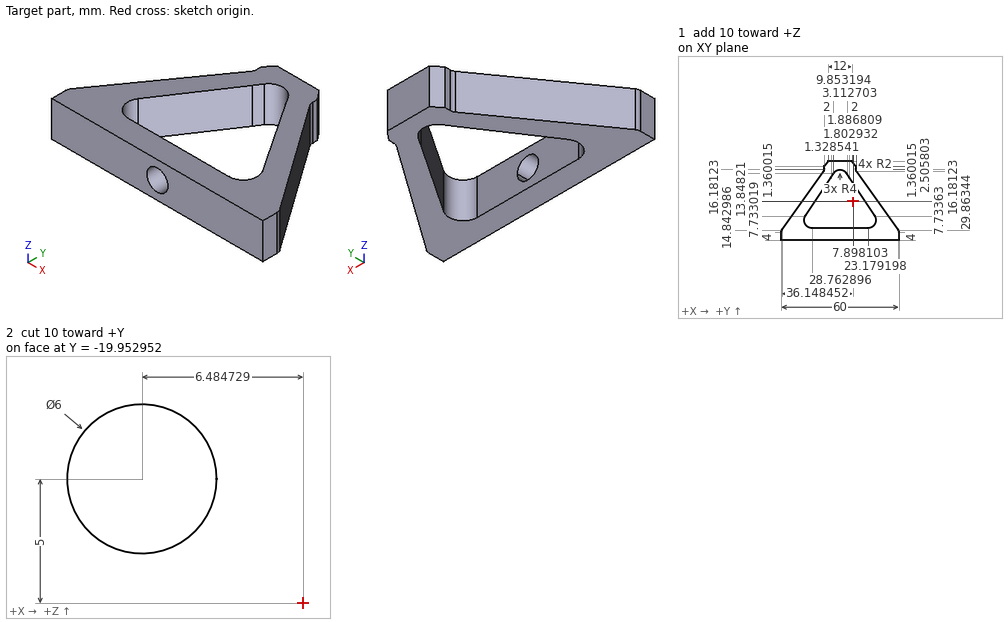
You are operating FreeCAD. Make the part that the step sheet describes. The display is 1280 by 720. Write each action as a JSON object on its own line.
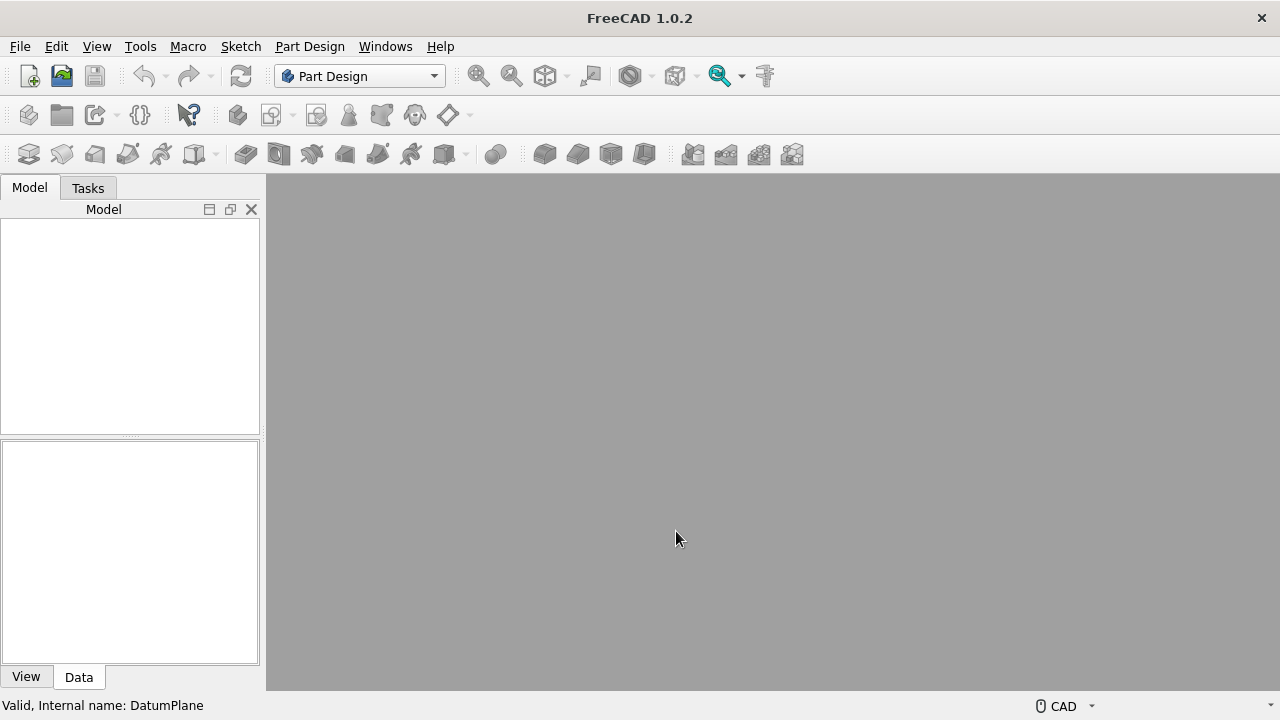
{"action": "left_click", "coordinate": [29, 76]}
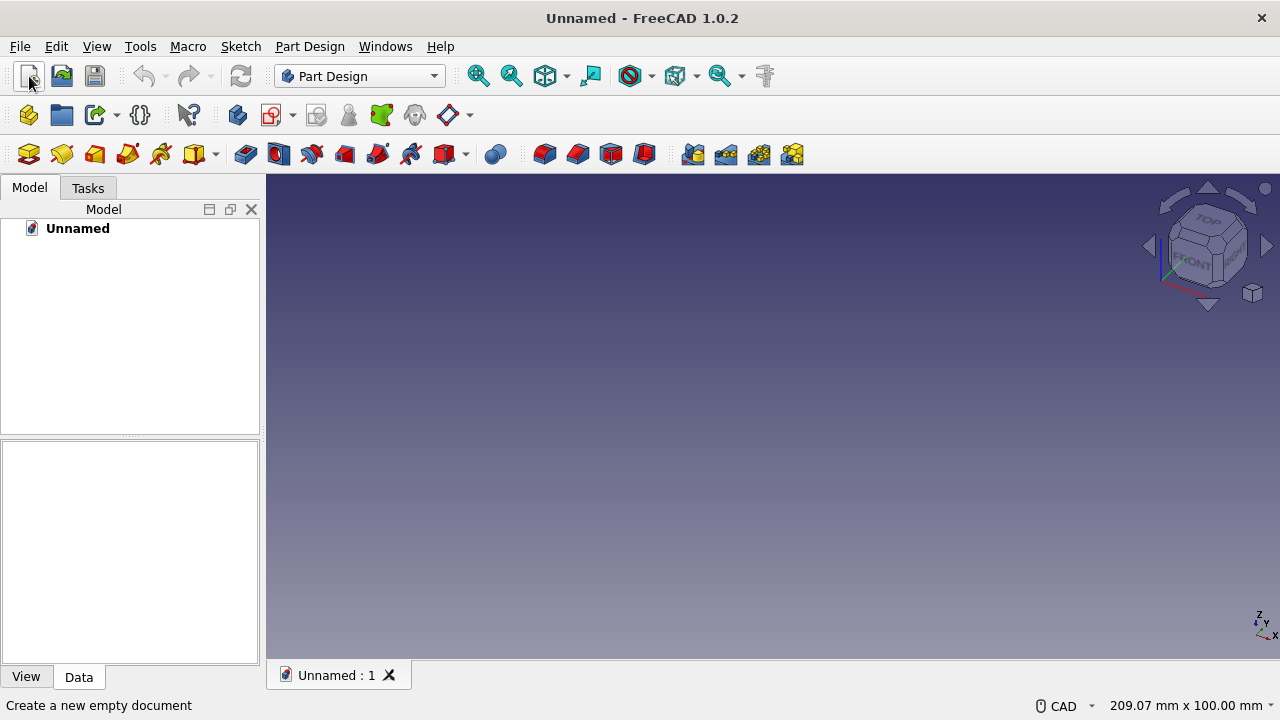
{"action": "left_click", "coordinate": [270, 116]}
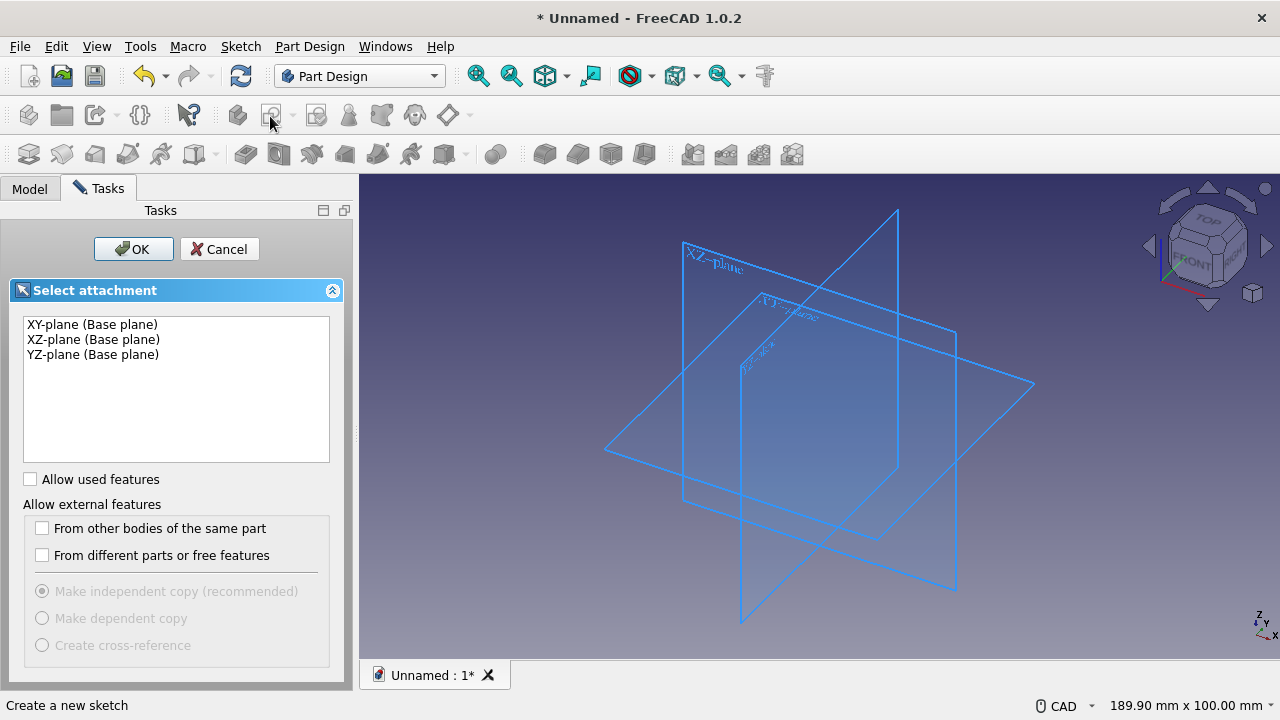
{"action": "left_click", "coordinate": [84, 324]}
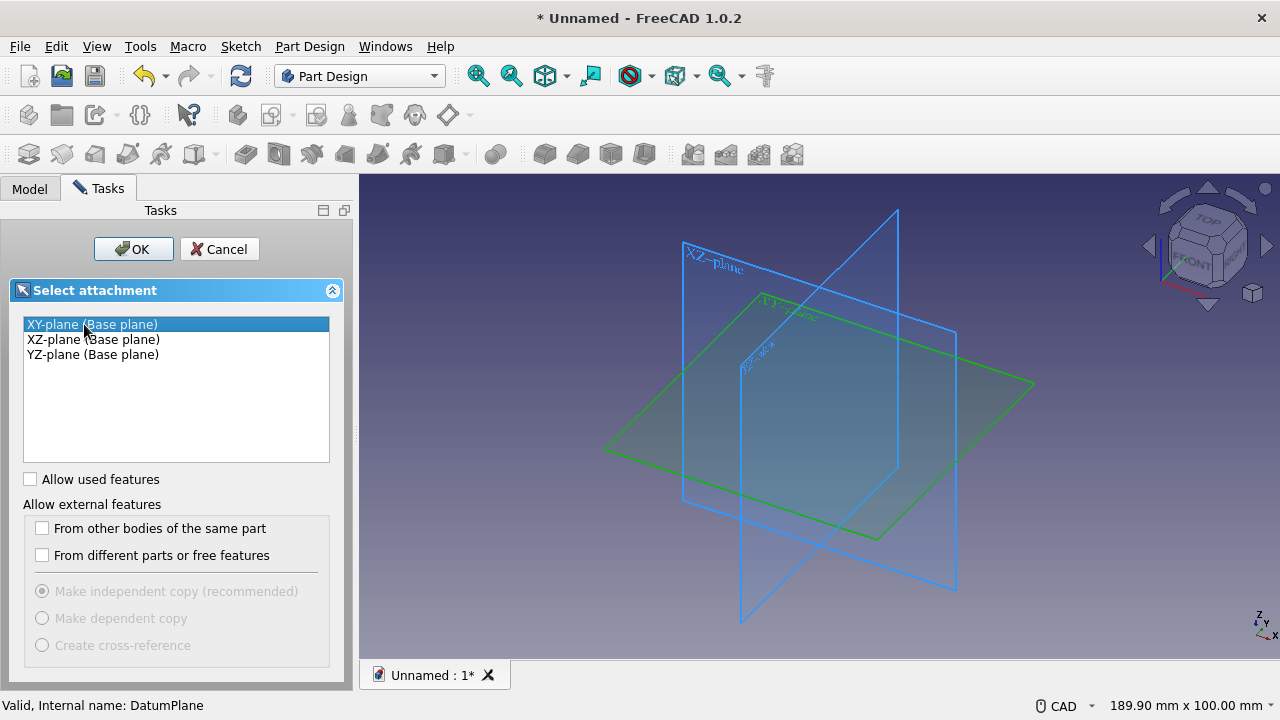
{"action": "left_click", "coordinate": [134, 249]}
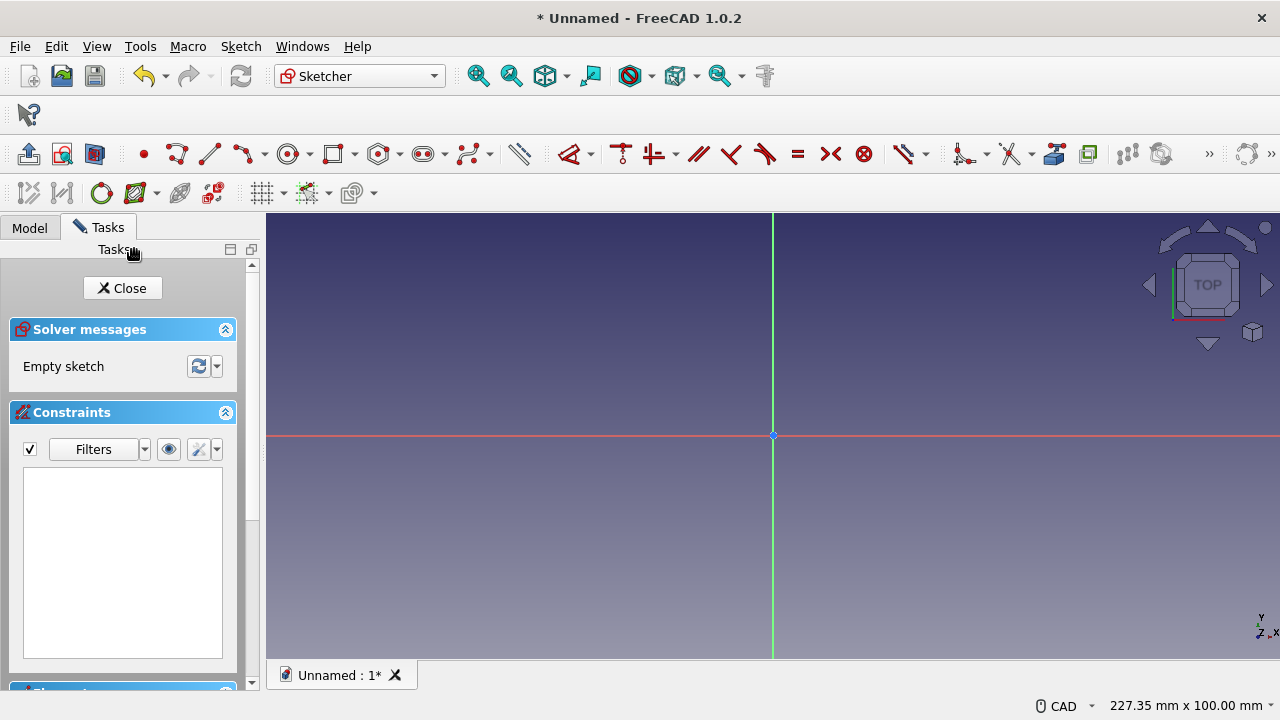
{"action": "scroll", "coordinate": [825, 435], "scroll_direction": "up", "scroll_amount": 2}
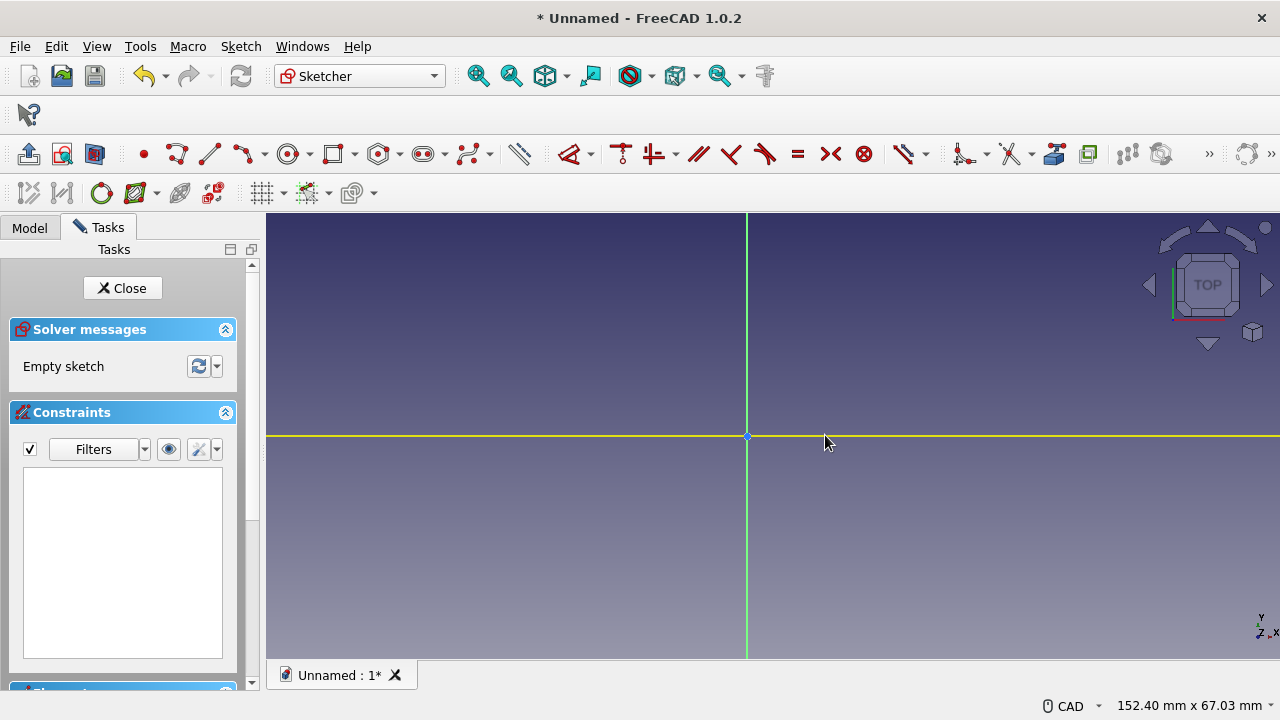
{"action": "left_click", "coordinate": [210, 154]}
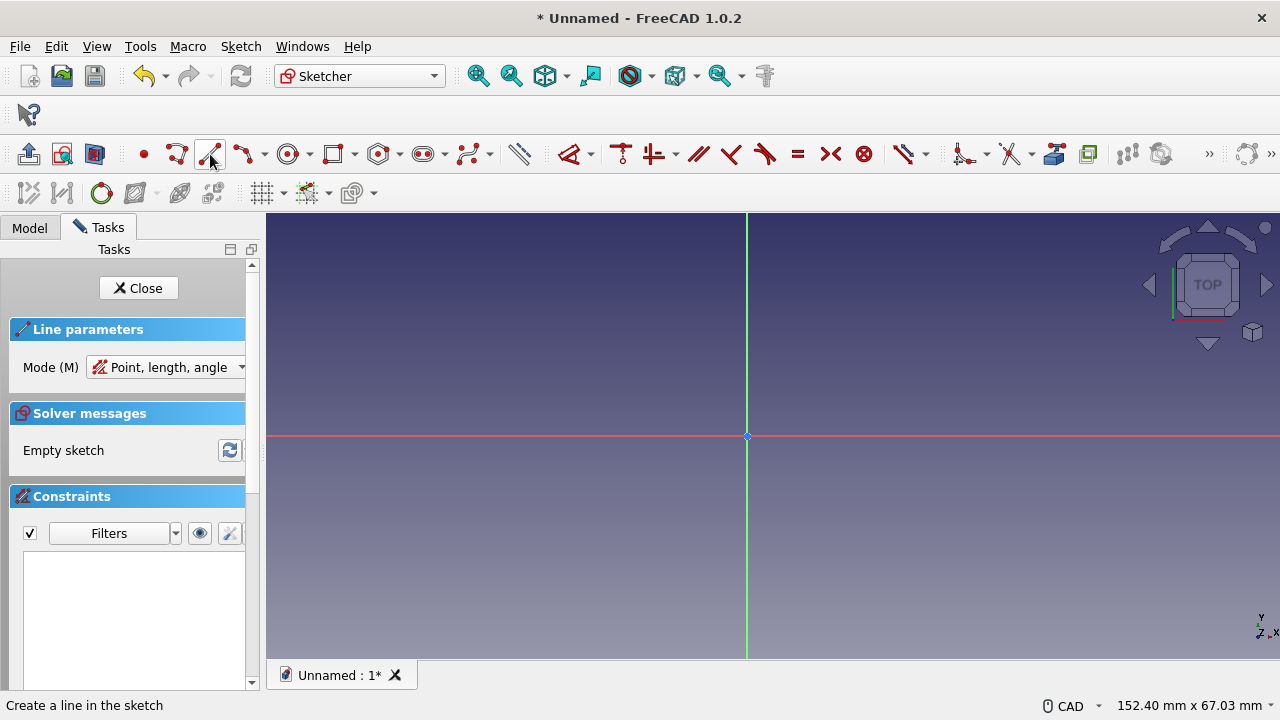
{"action": "left_click", "coordinate": [901, 535]}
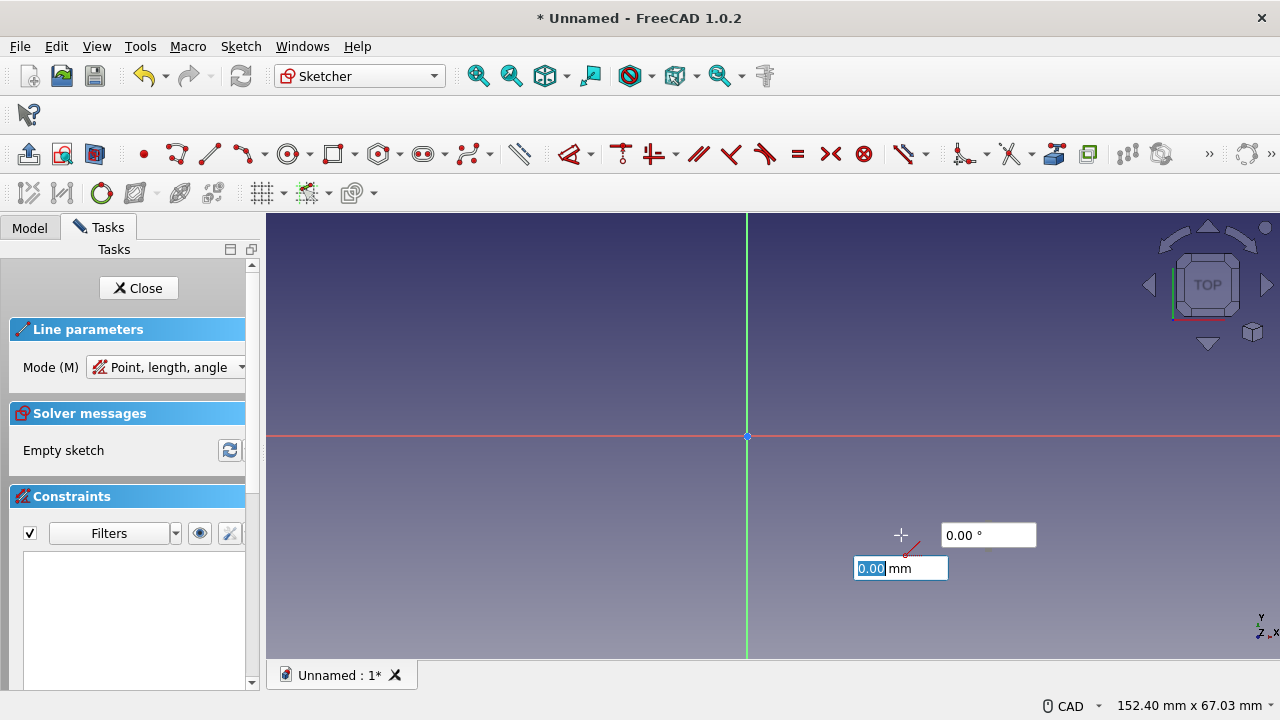
{"action": "scroll", "coordinate": [760, 336], "scroll_direction": "up", "scroll_amount": 2}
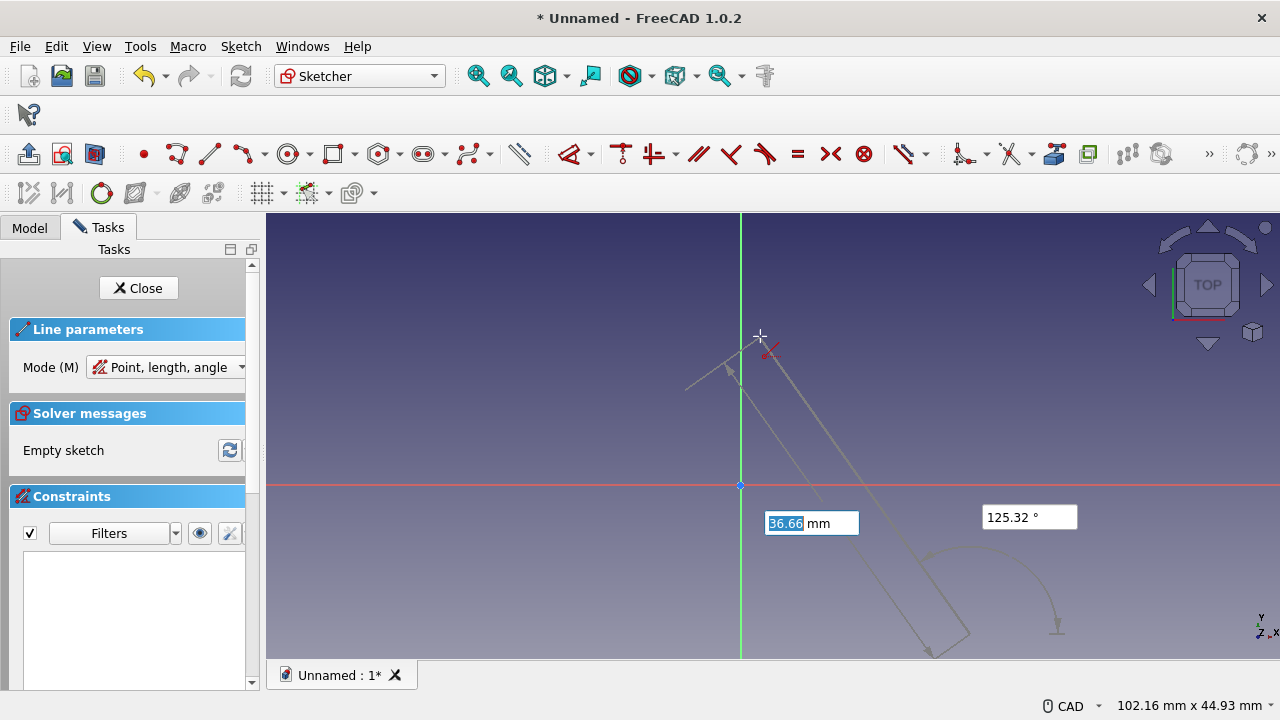
{"action": "left_click", "coordinate": [759, 336]}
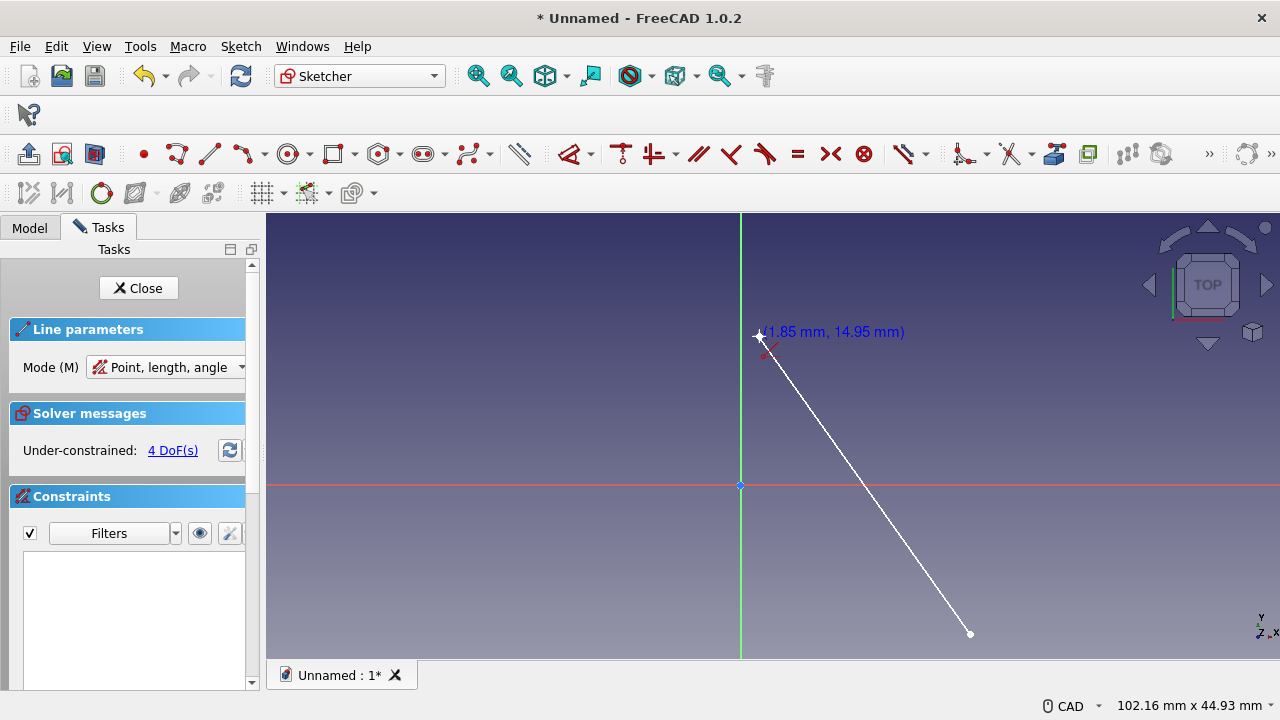
{"action": "left_click", "coordinate": [177, 154]}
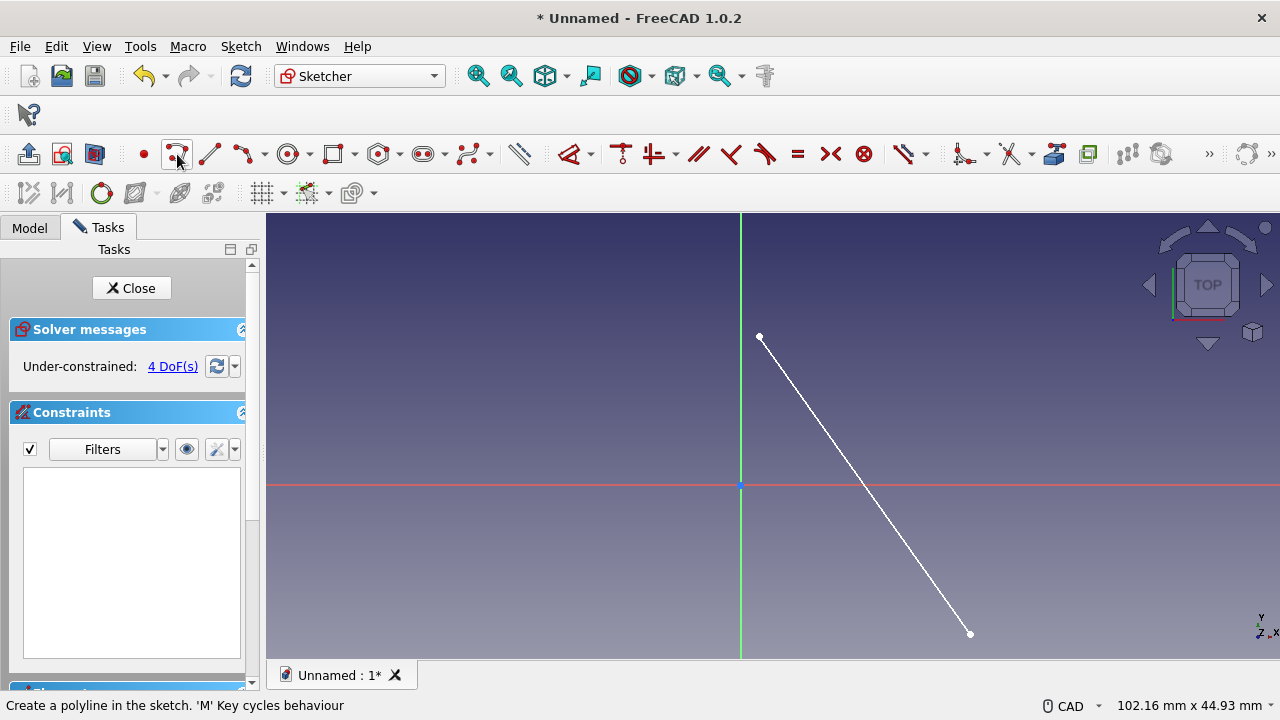
{"action": "scroll", "coordinate": [756, 325], "scroll_direction": "up", "scroll_amount": 2}